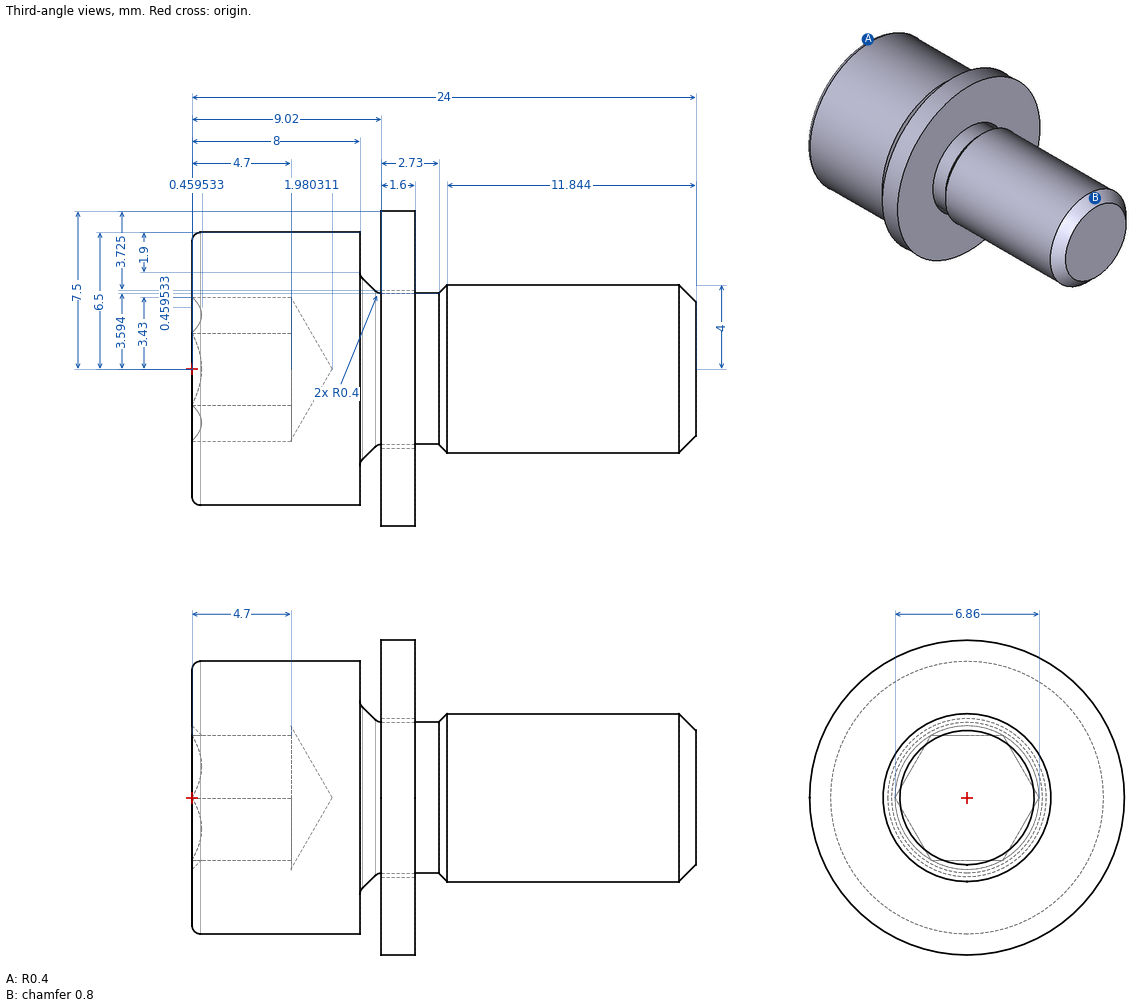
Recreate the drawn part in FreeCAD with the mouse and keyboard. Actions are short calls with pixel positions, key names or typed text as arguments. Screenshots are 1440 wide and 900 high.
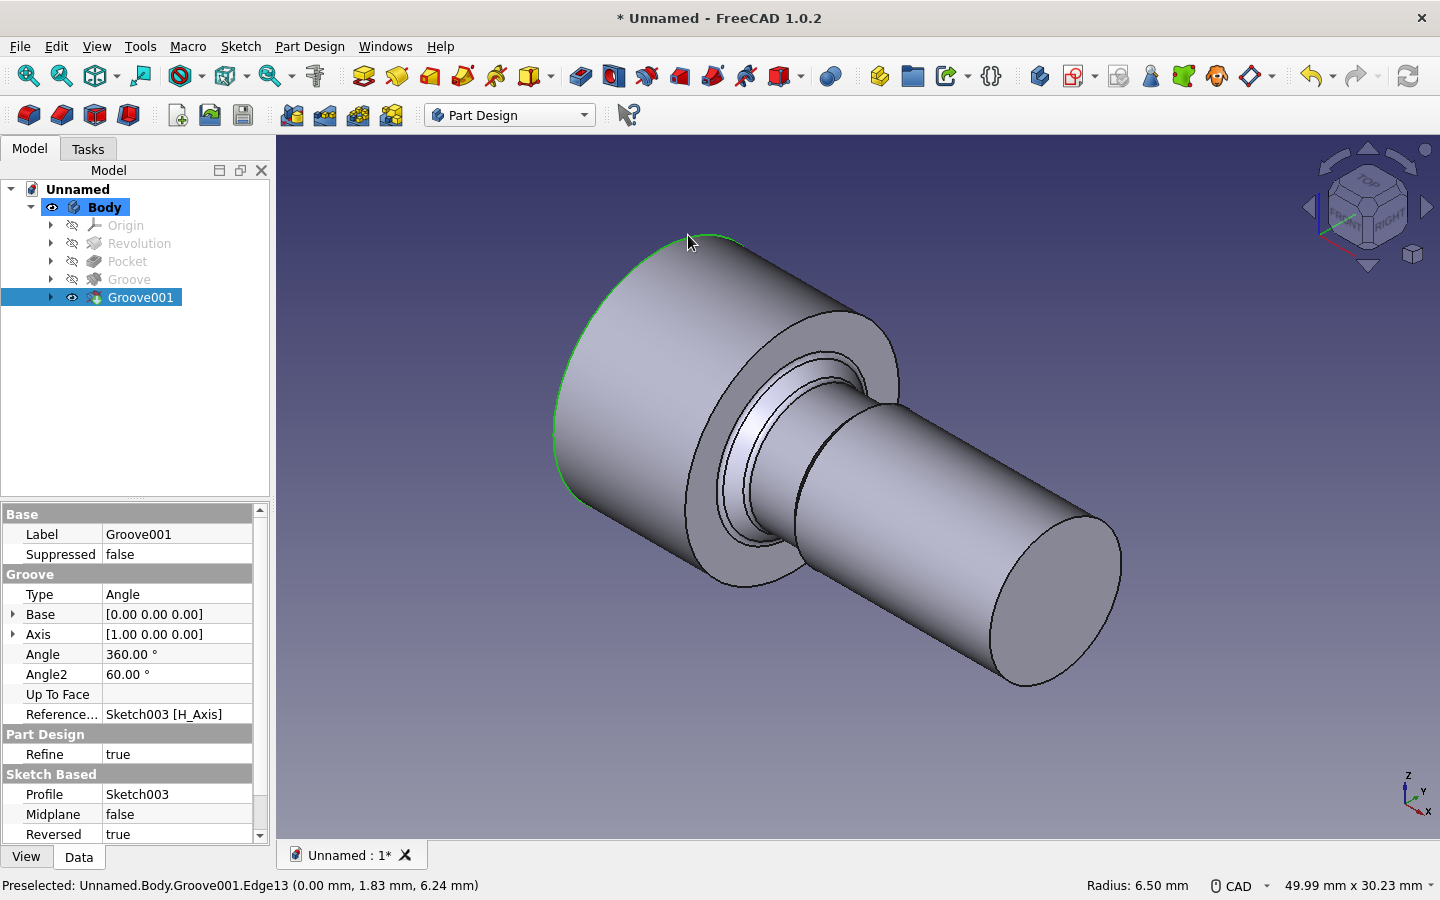
click(29, 116)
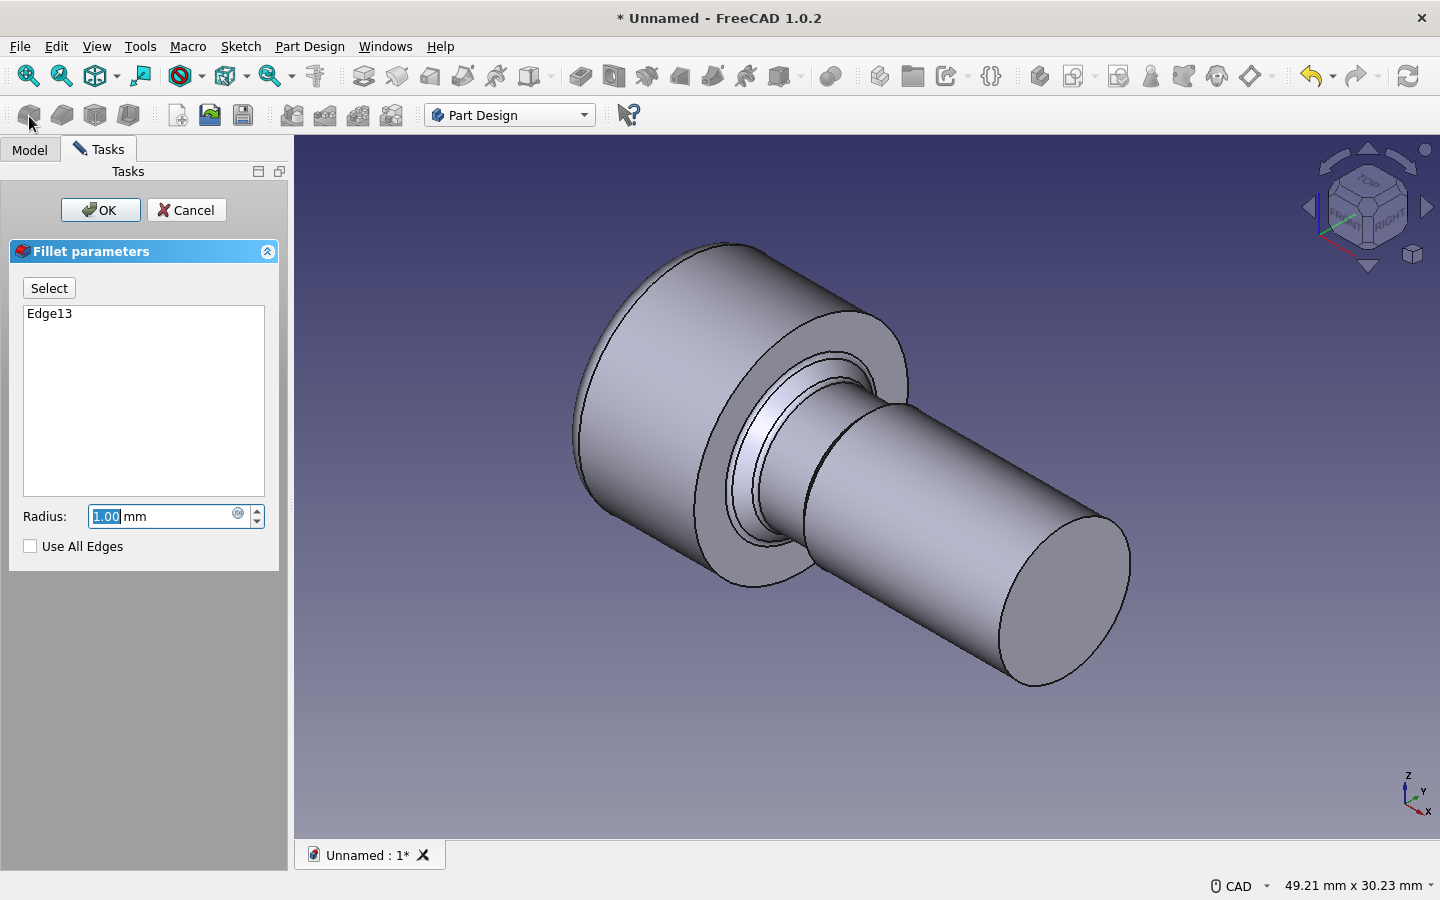
text(0.4)
key(Tab)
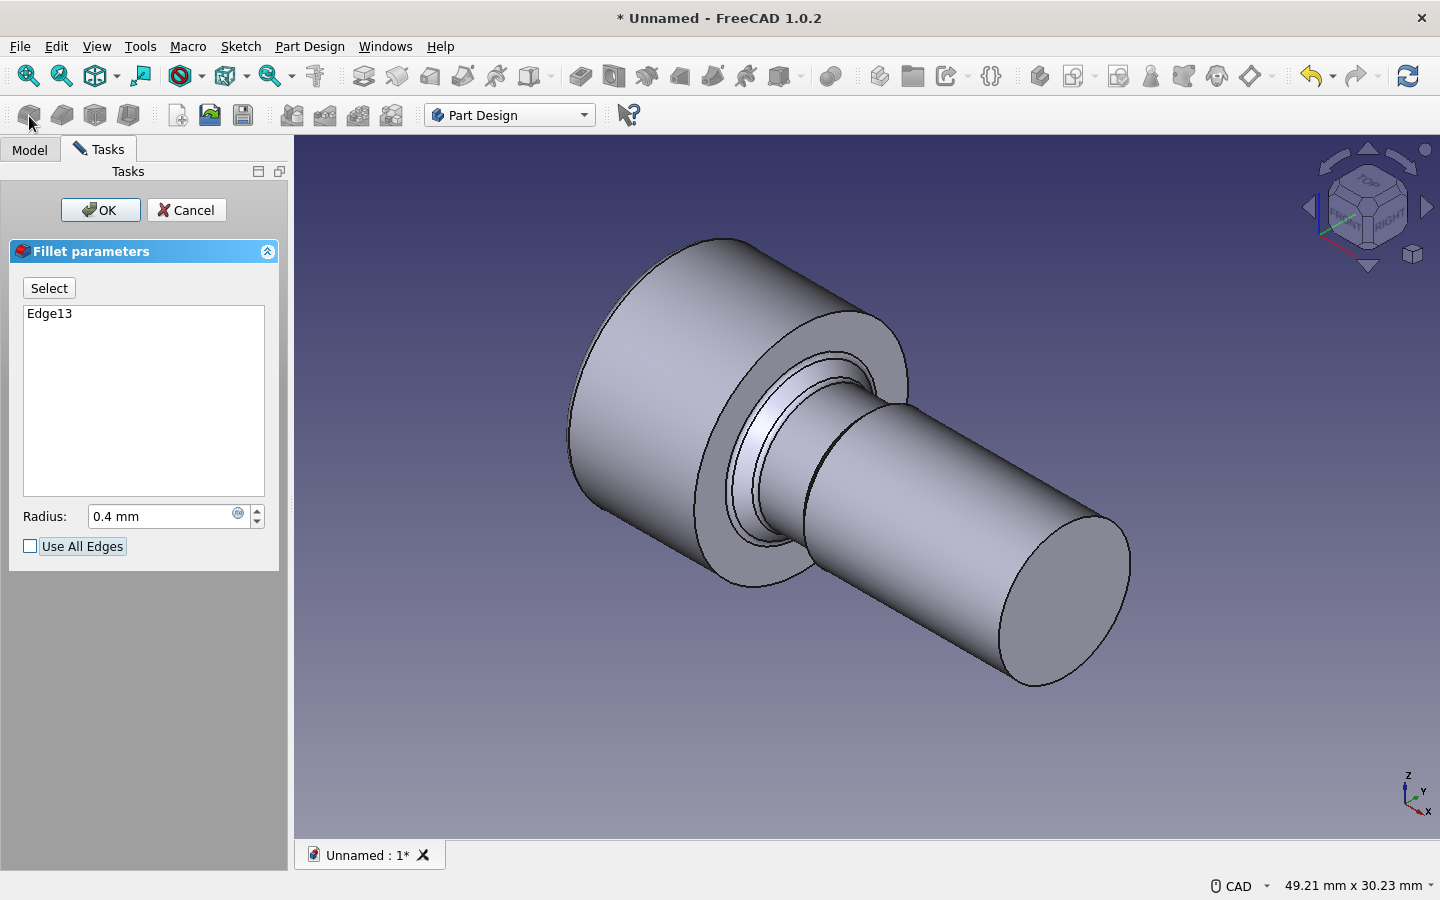
click(101, 210)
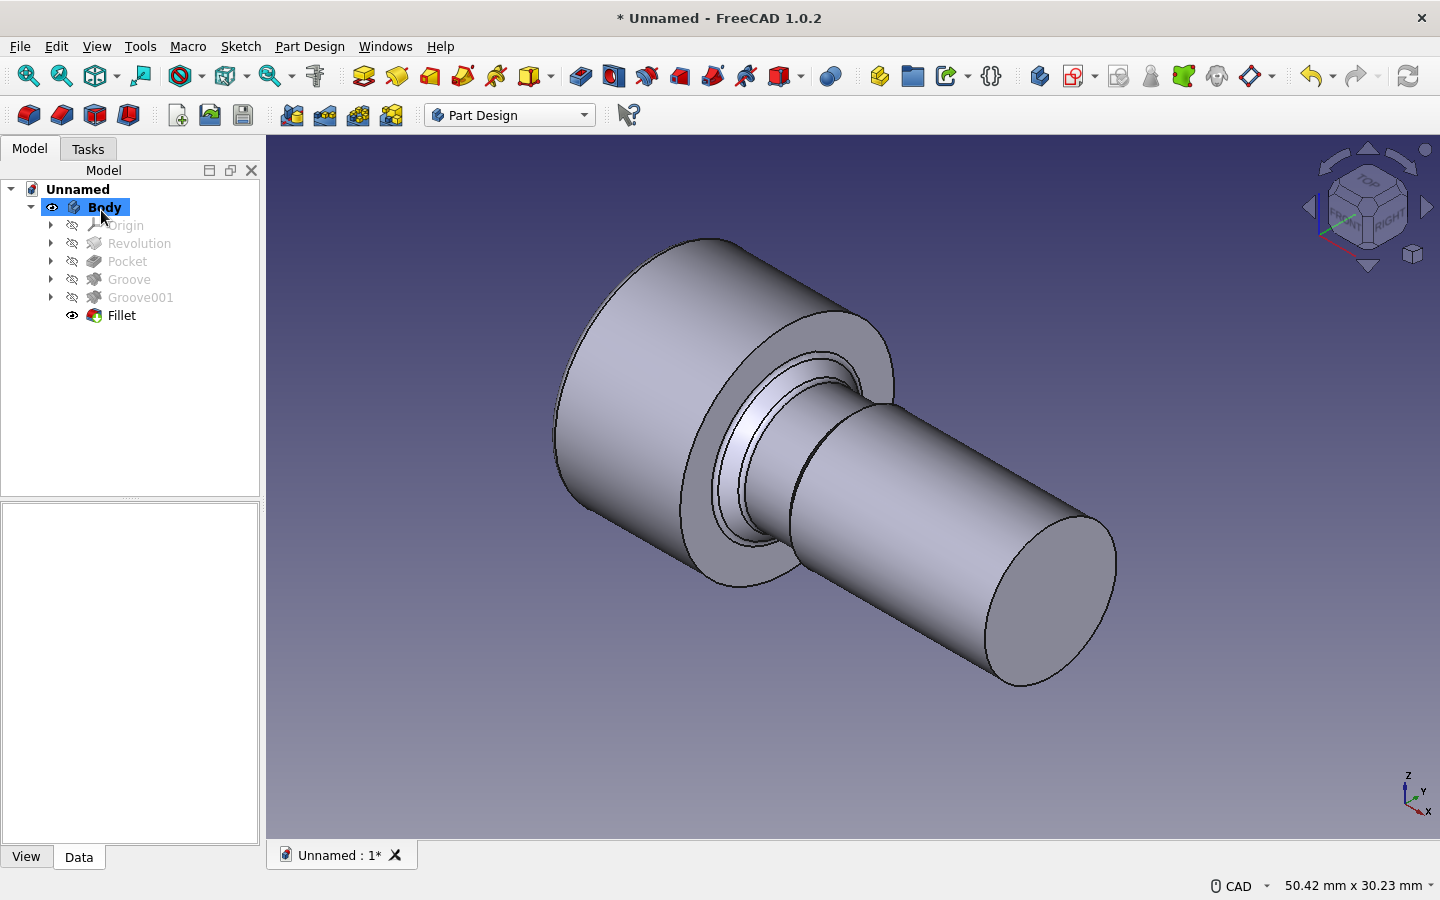
click(985, 638)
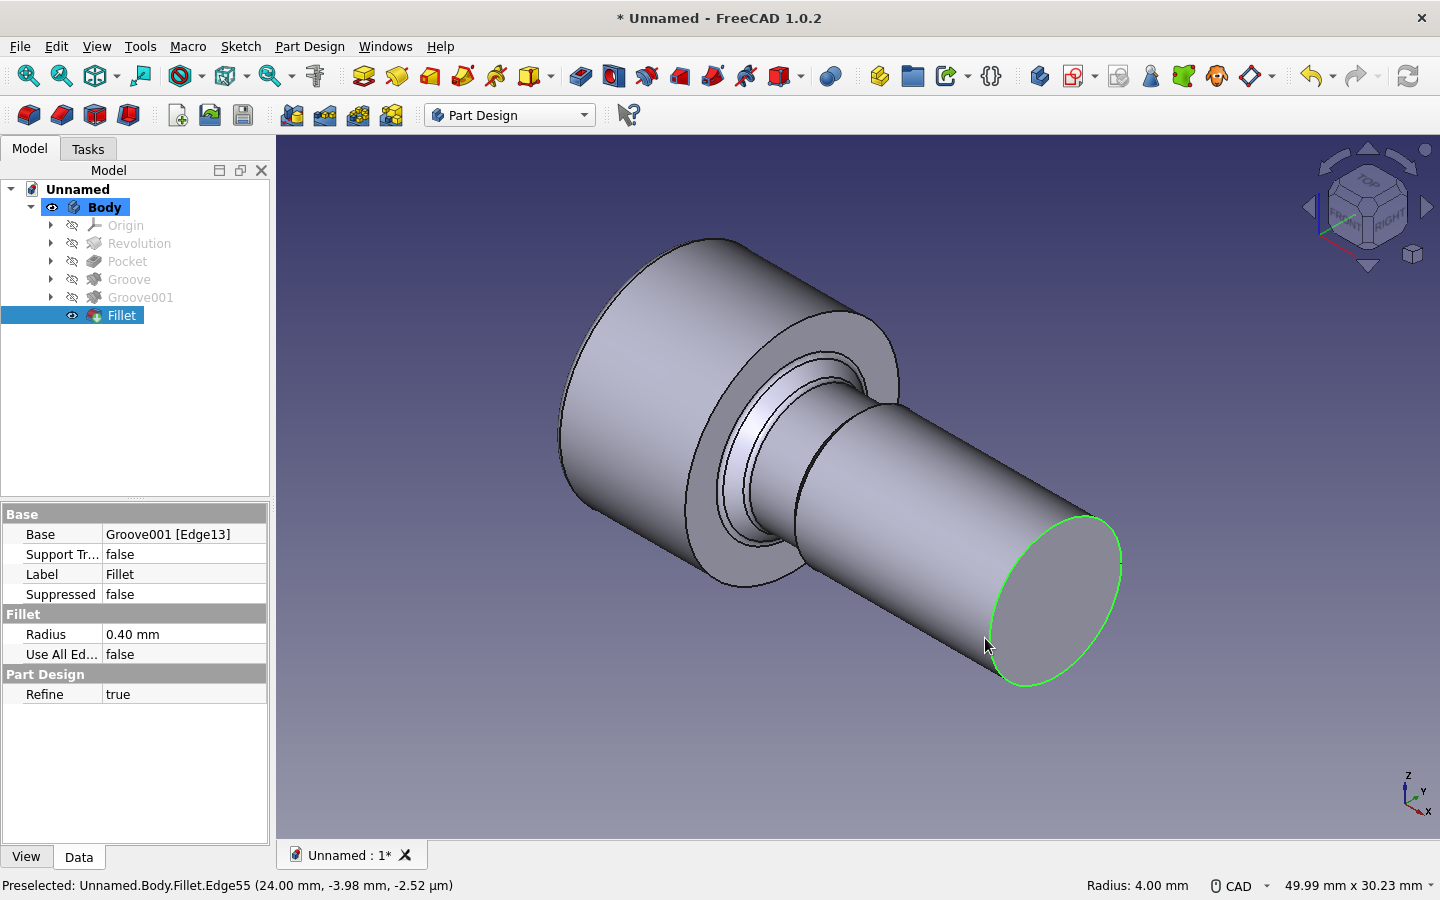
click(62, 116)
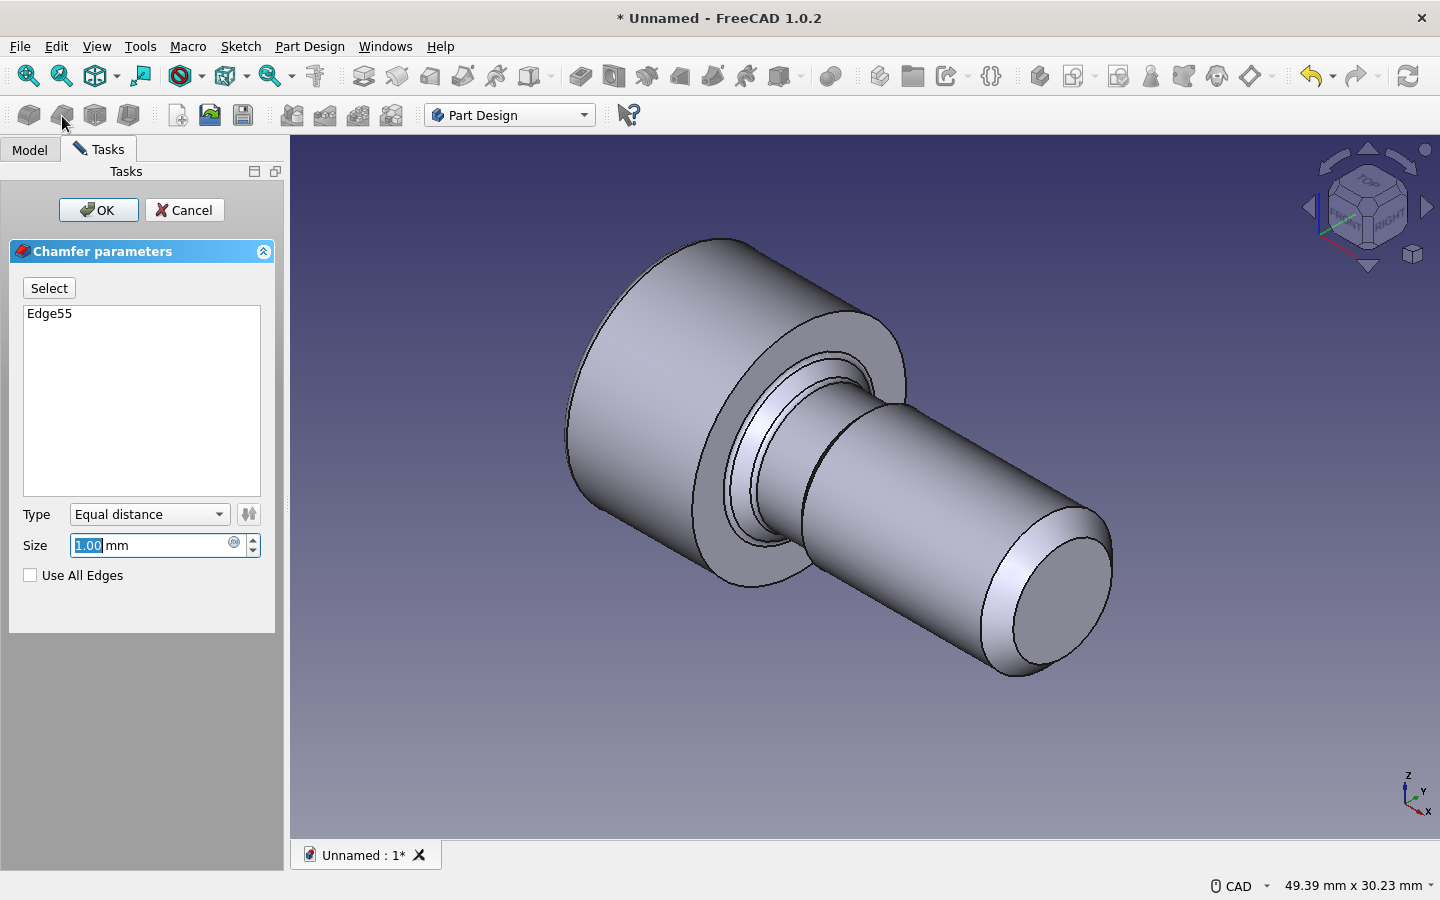
text(0.8)
key(Tab)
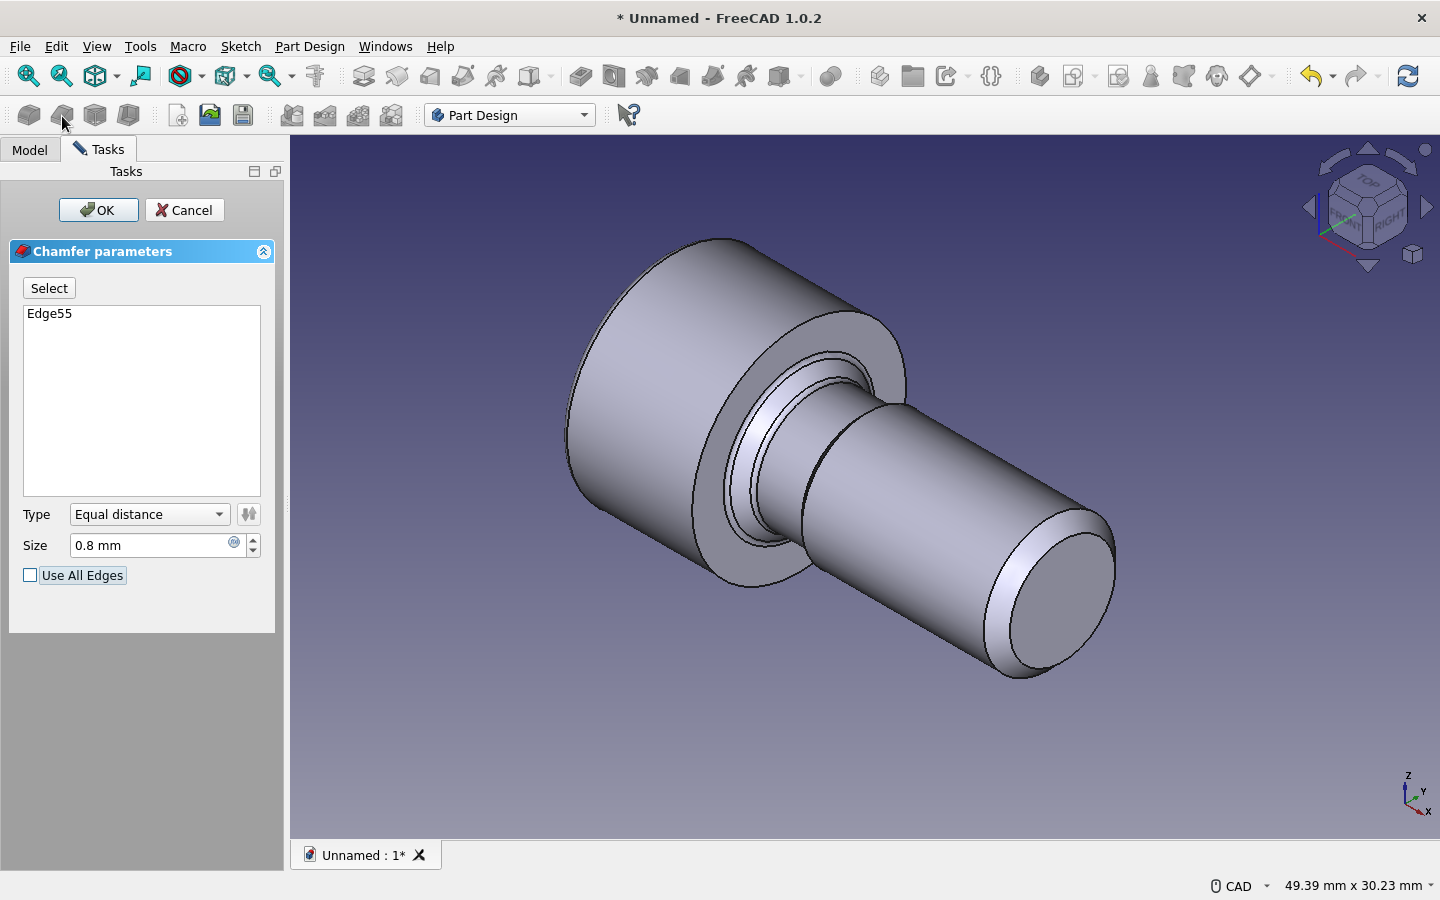
click(99, 210)